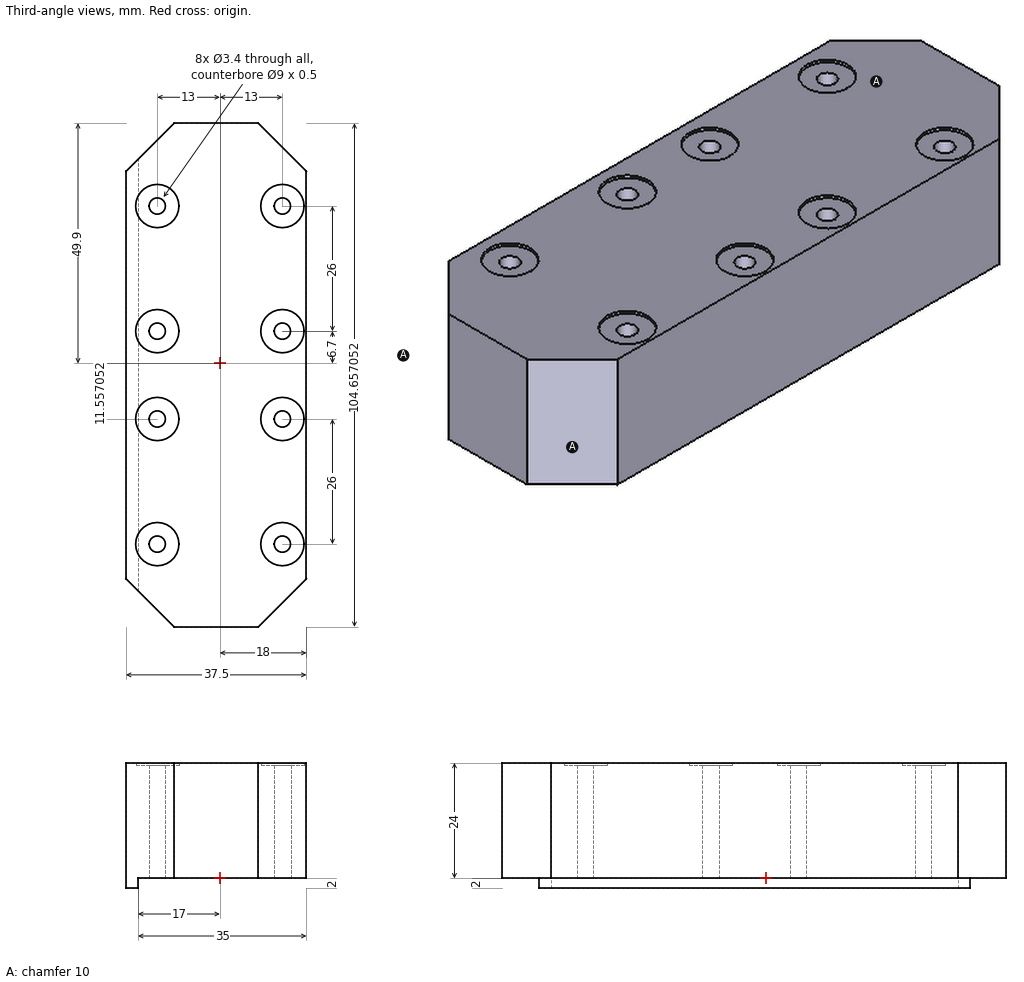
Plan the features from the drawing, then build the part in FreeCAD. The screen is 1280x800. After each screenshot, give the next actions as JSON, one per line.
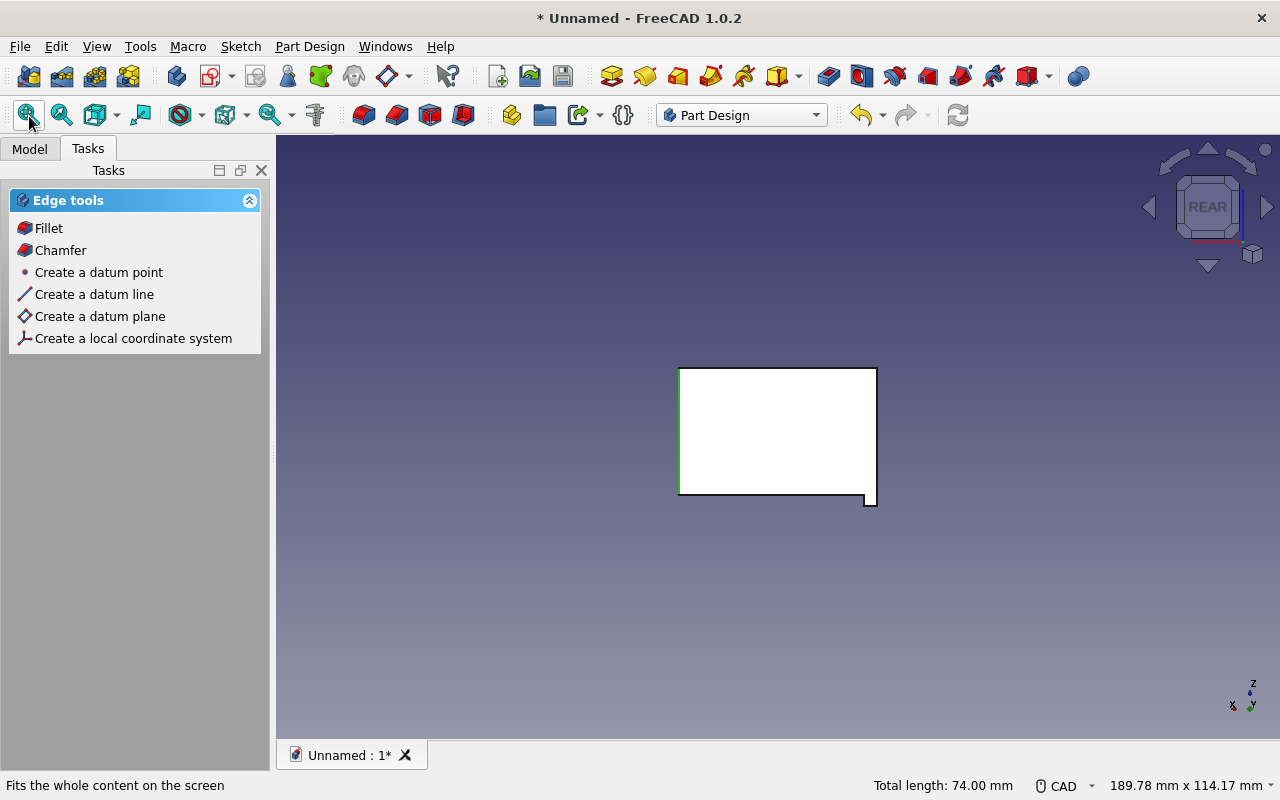
{"action": "left_click", "coordinate": [877, 436], "text": "ctrl"}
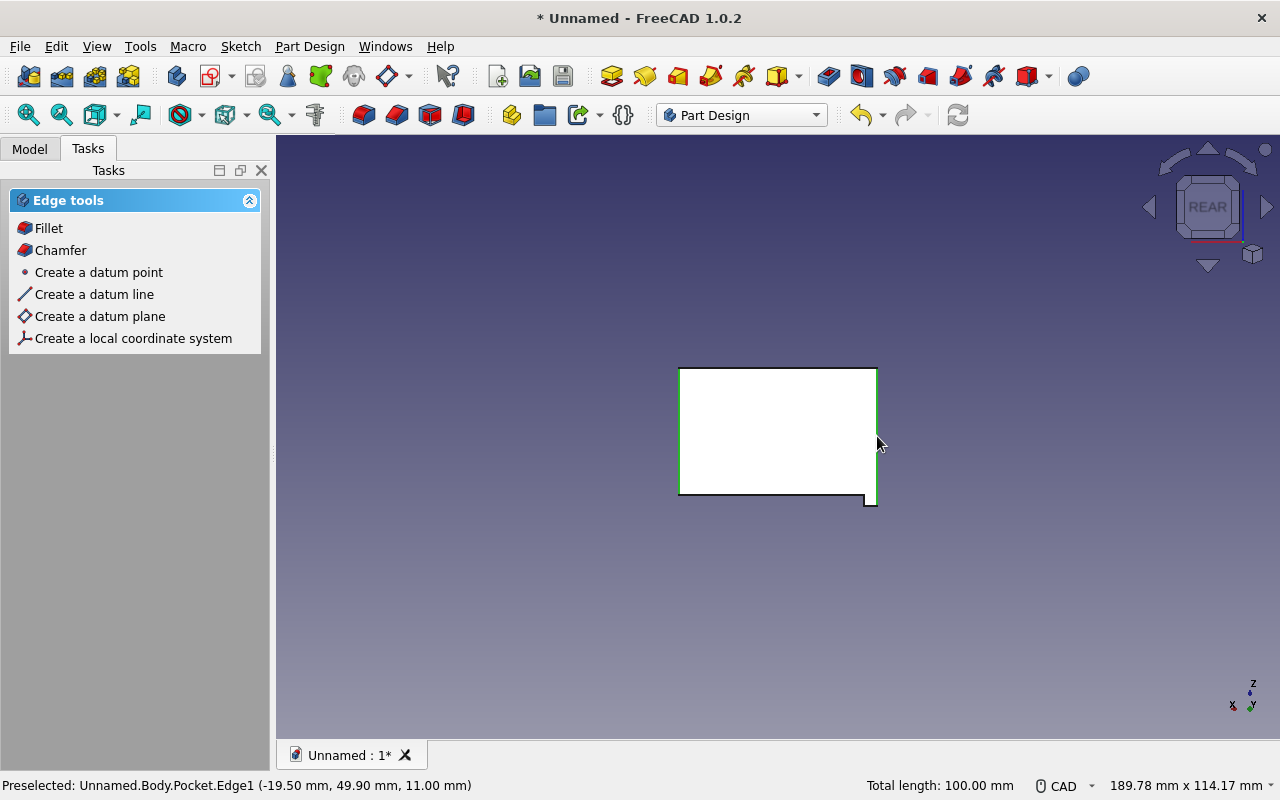
{"action": "left_click", "coordinate": [397, 116]}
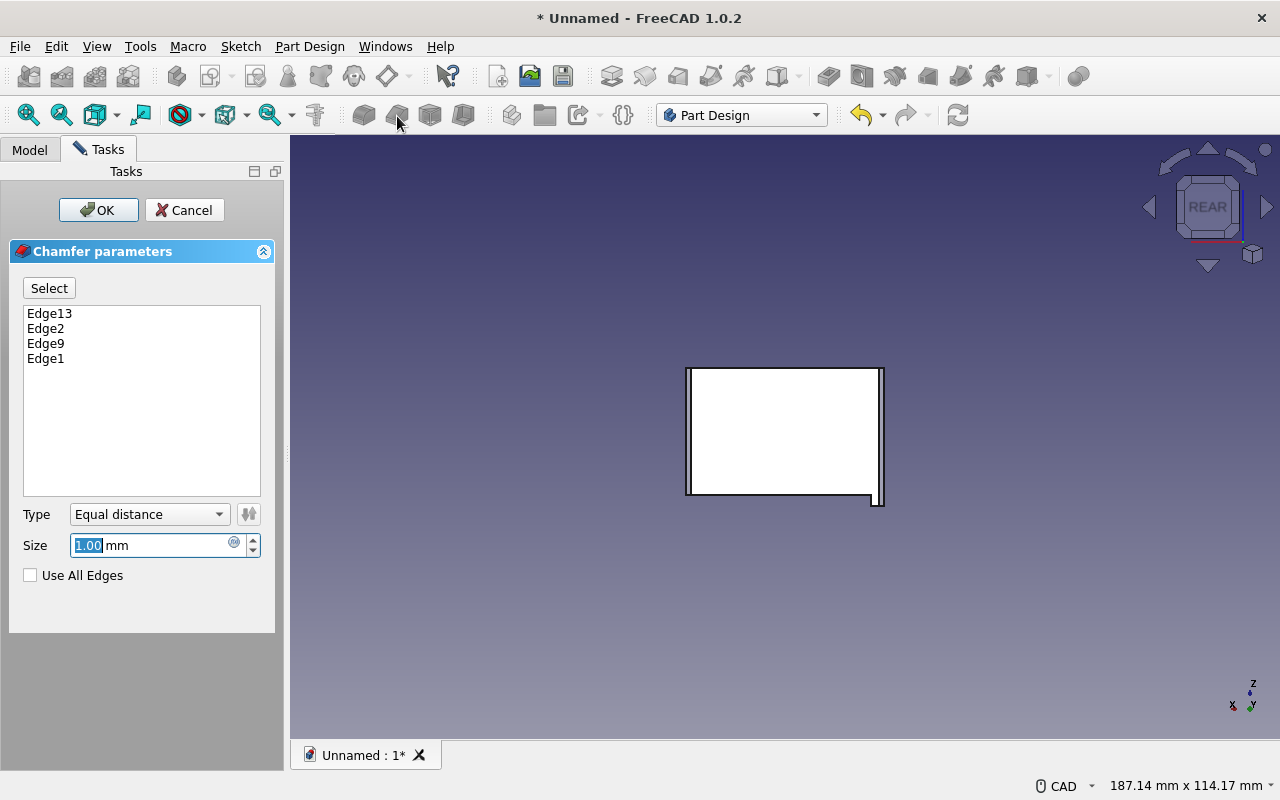
{"action": "type", "text": "10"}
{"action": "key", "text": "Tab"}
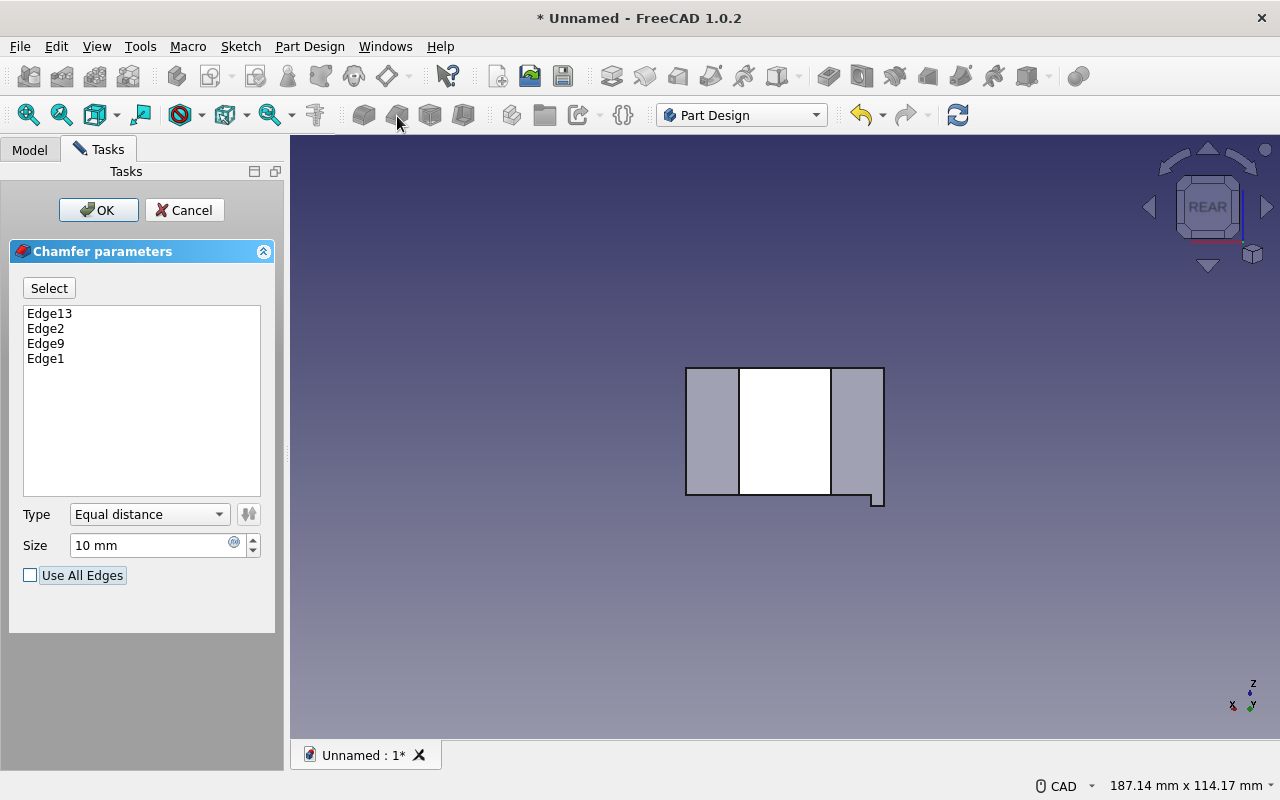
{"action": "left_click", "coordinate": [99, 210]}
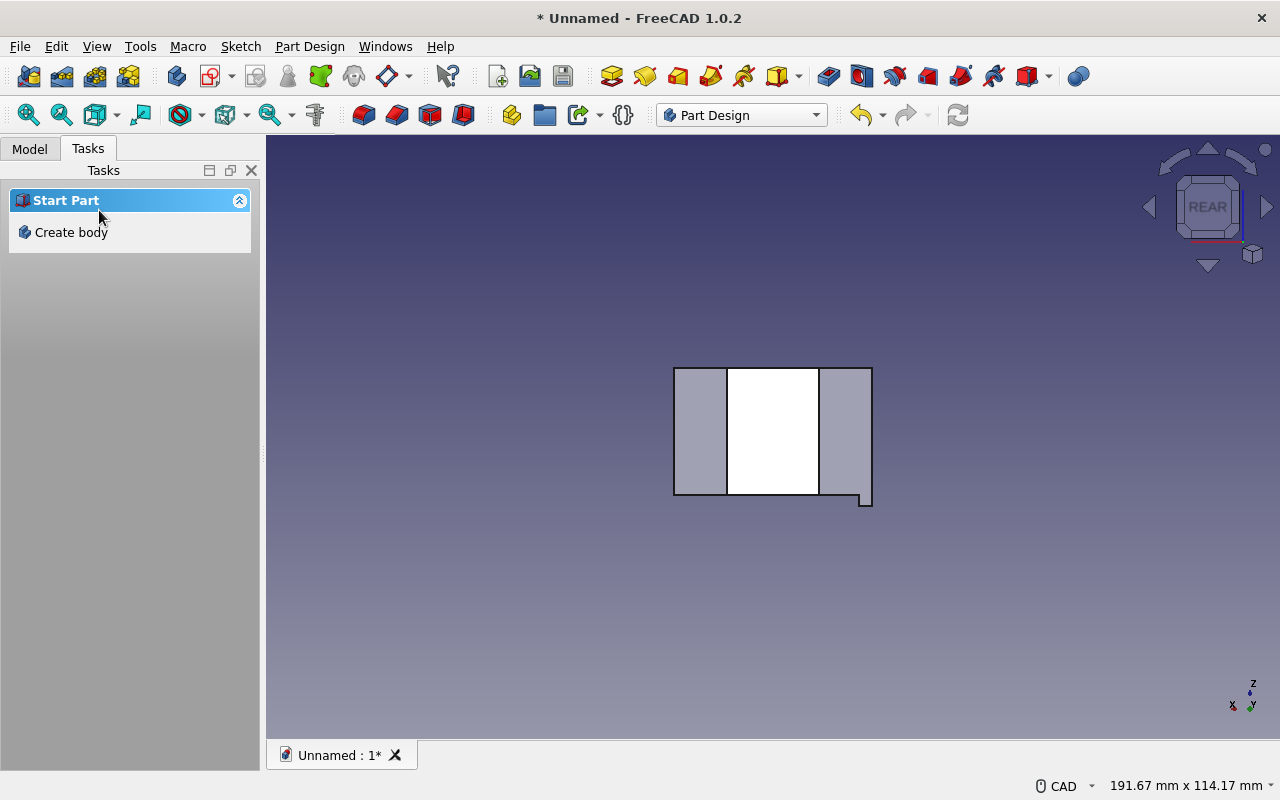
{"action": "left_click", "coordinate": [29, 116]}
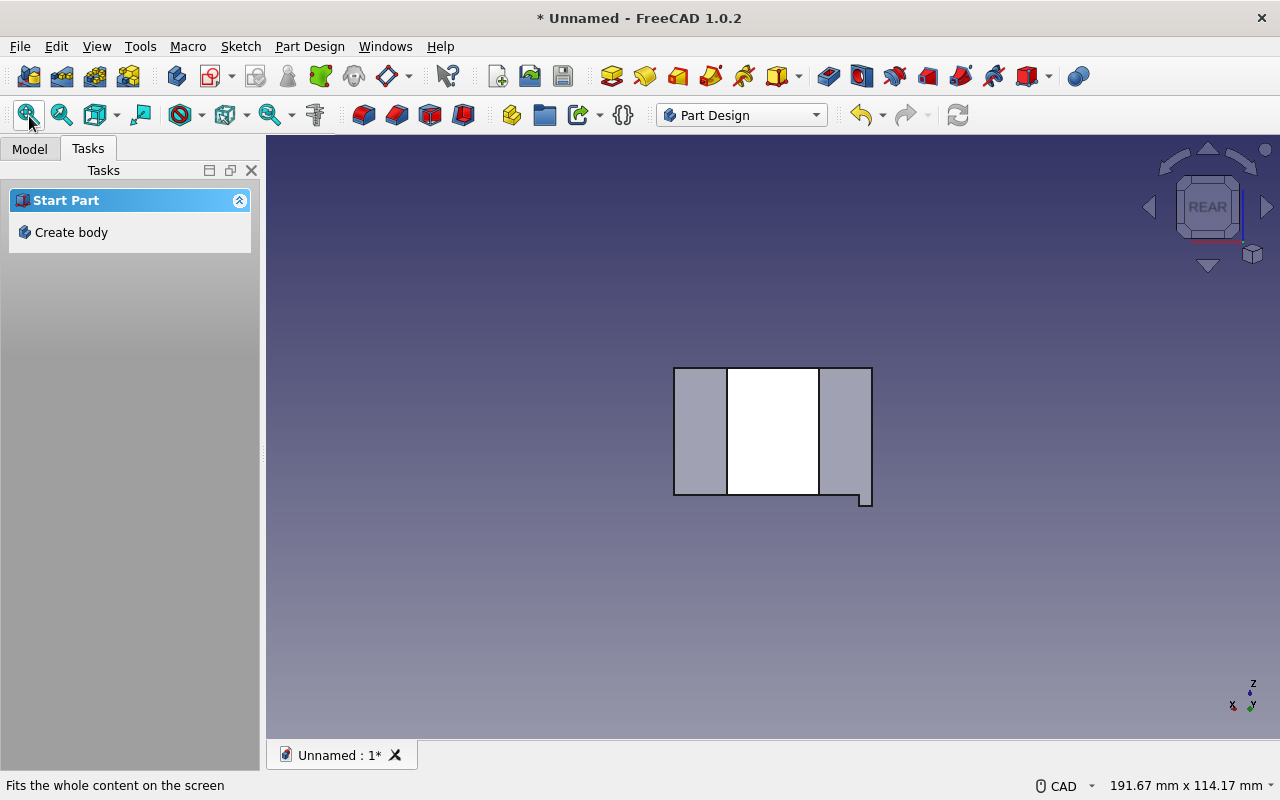
{"action": "key", "text": "0"}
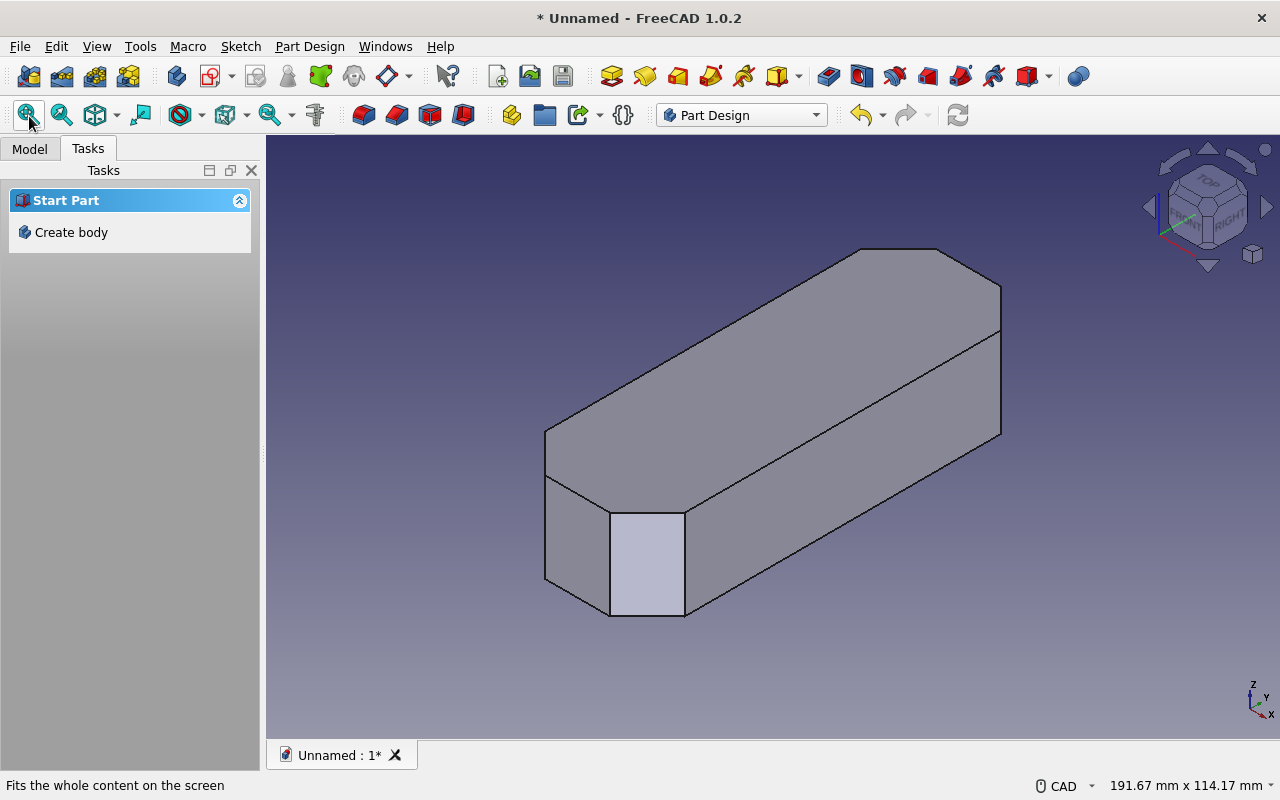
{"action": "left_click", "coordinate": [885, 315]}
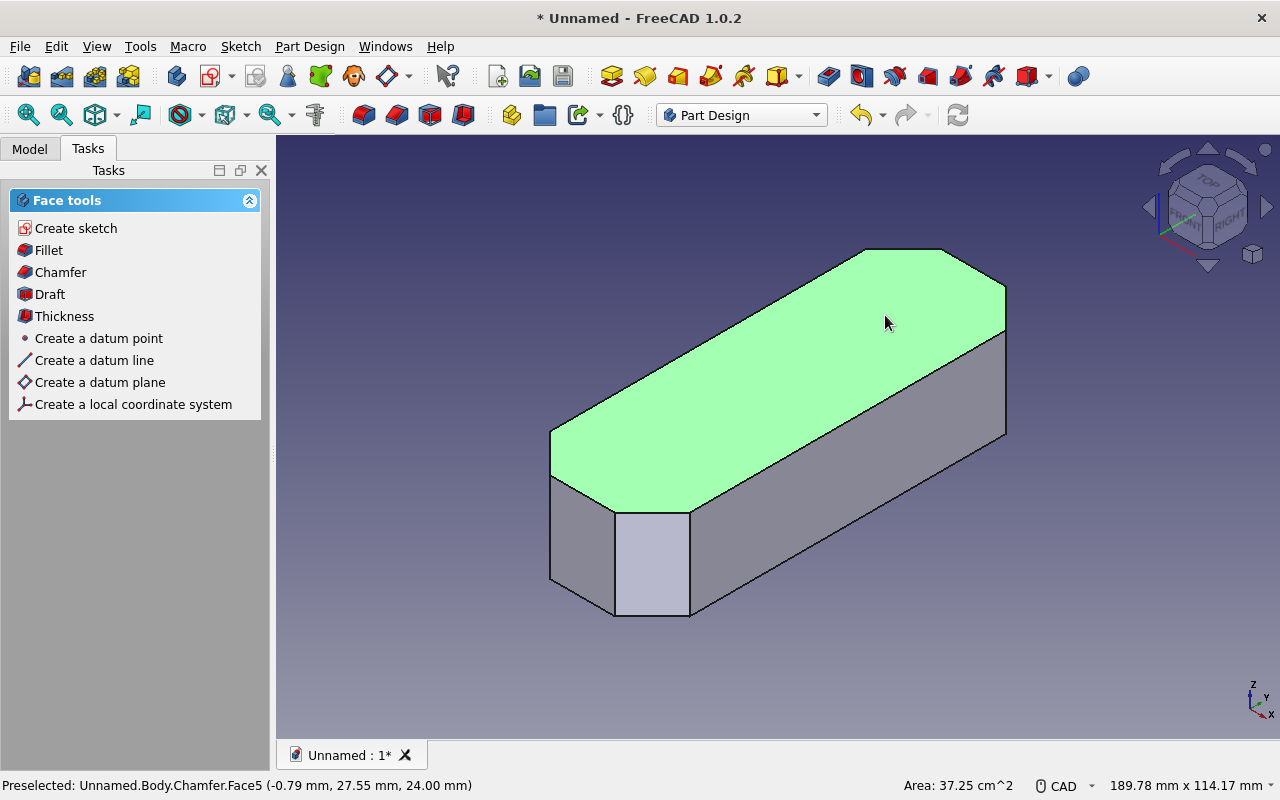
{"action": "left_click", "coordinate": [210, 76]}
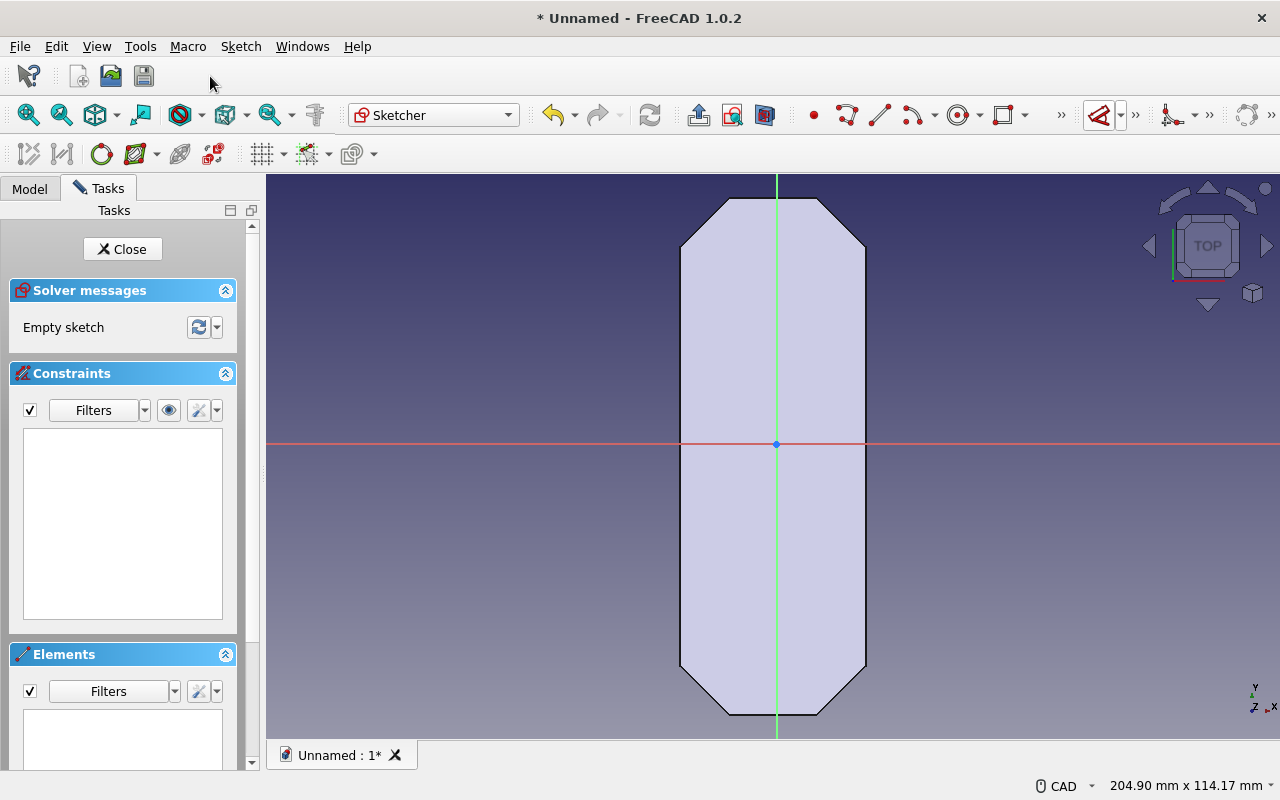
{"action": "left_click", "coordinate": [958, 116]}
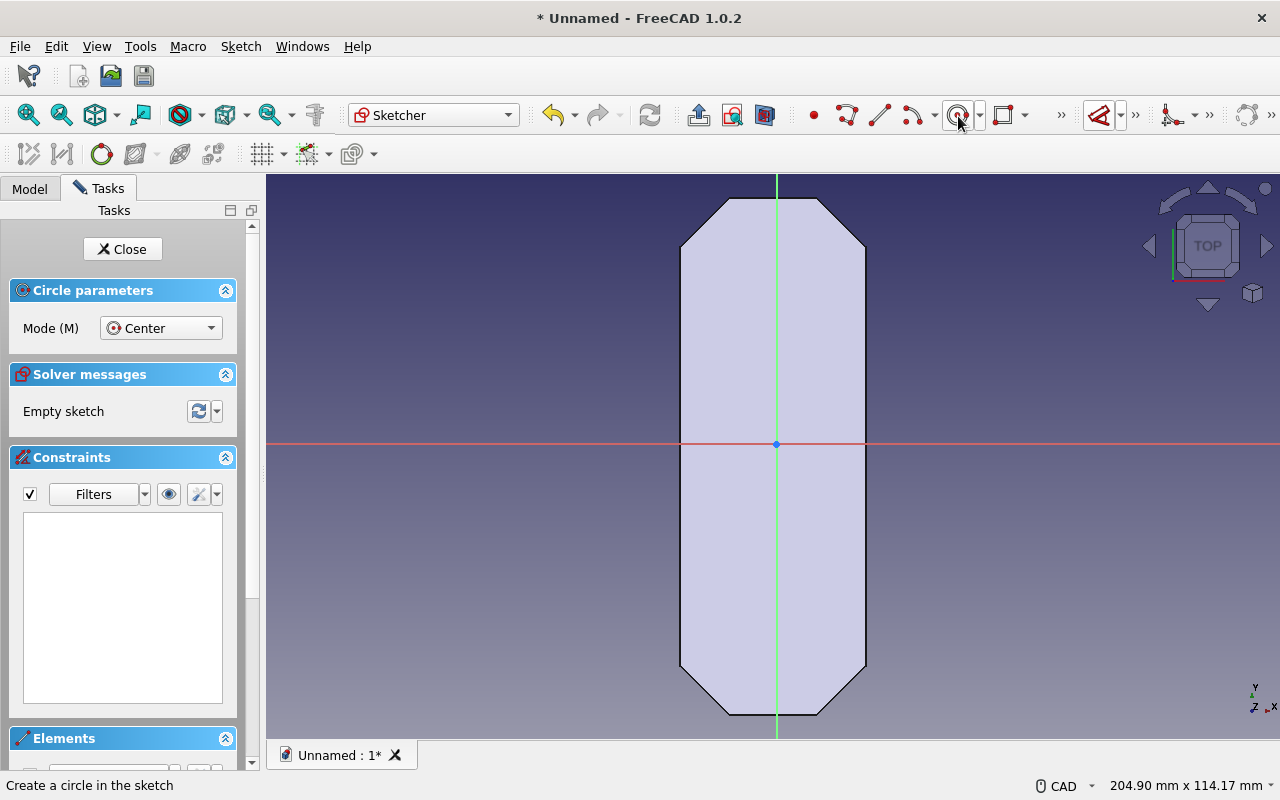
{"action": "scroll", "coordinate": [712, 283], "scroll_direction": "up", "scroll_amount": 5}